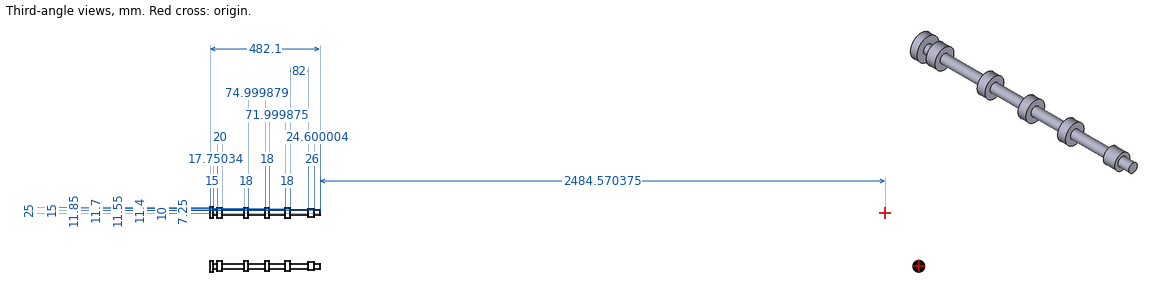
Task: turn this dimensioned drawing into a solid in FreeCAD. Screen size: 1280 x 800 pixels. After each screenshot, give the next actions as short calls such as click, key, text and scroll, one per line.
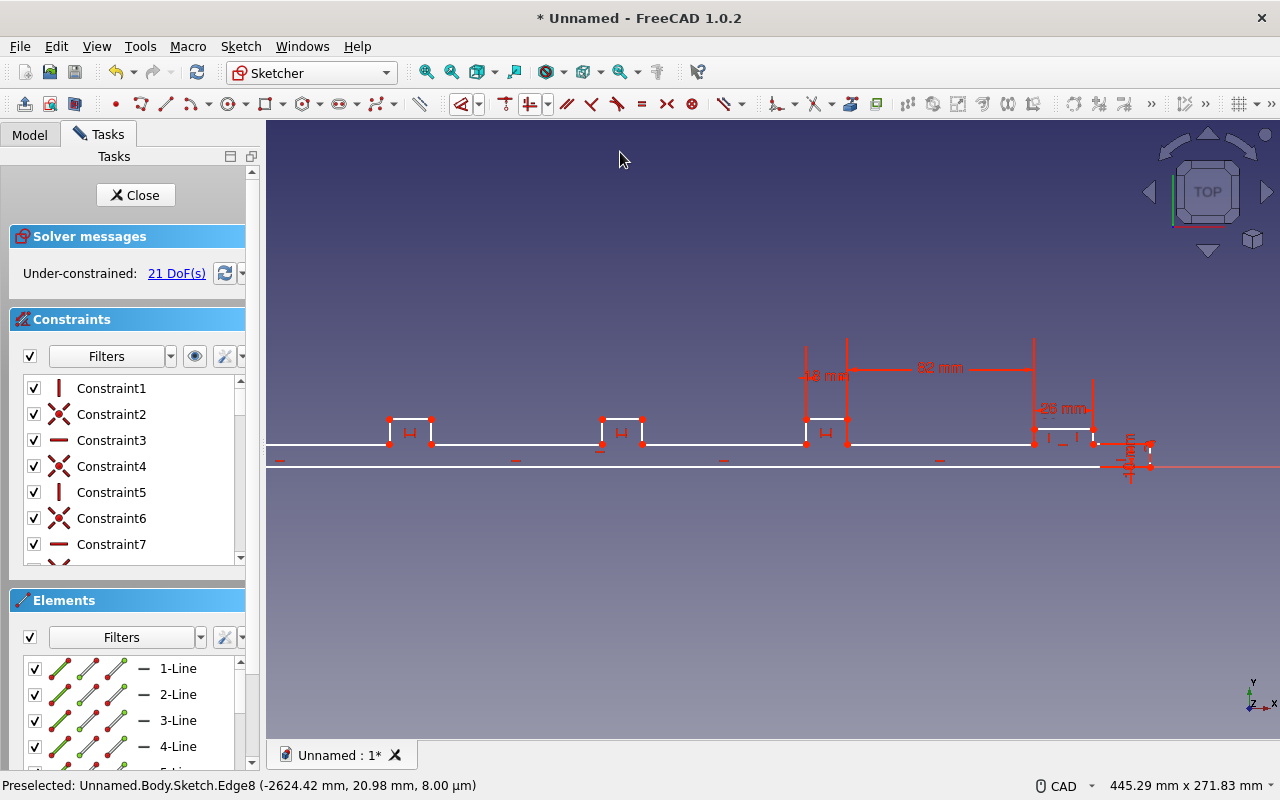
click(630, 419)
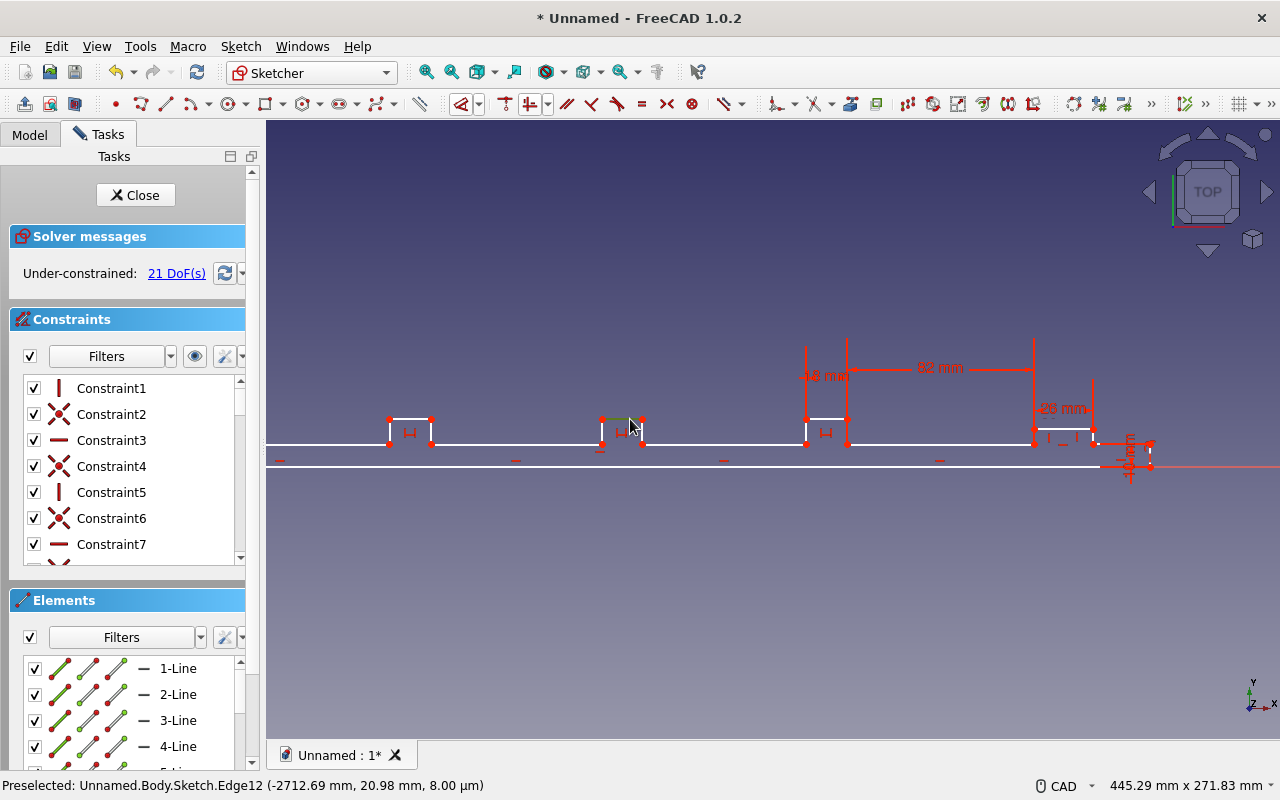
click(478, 104)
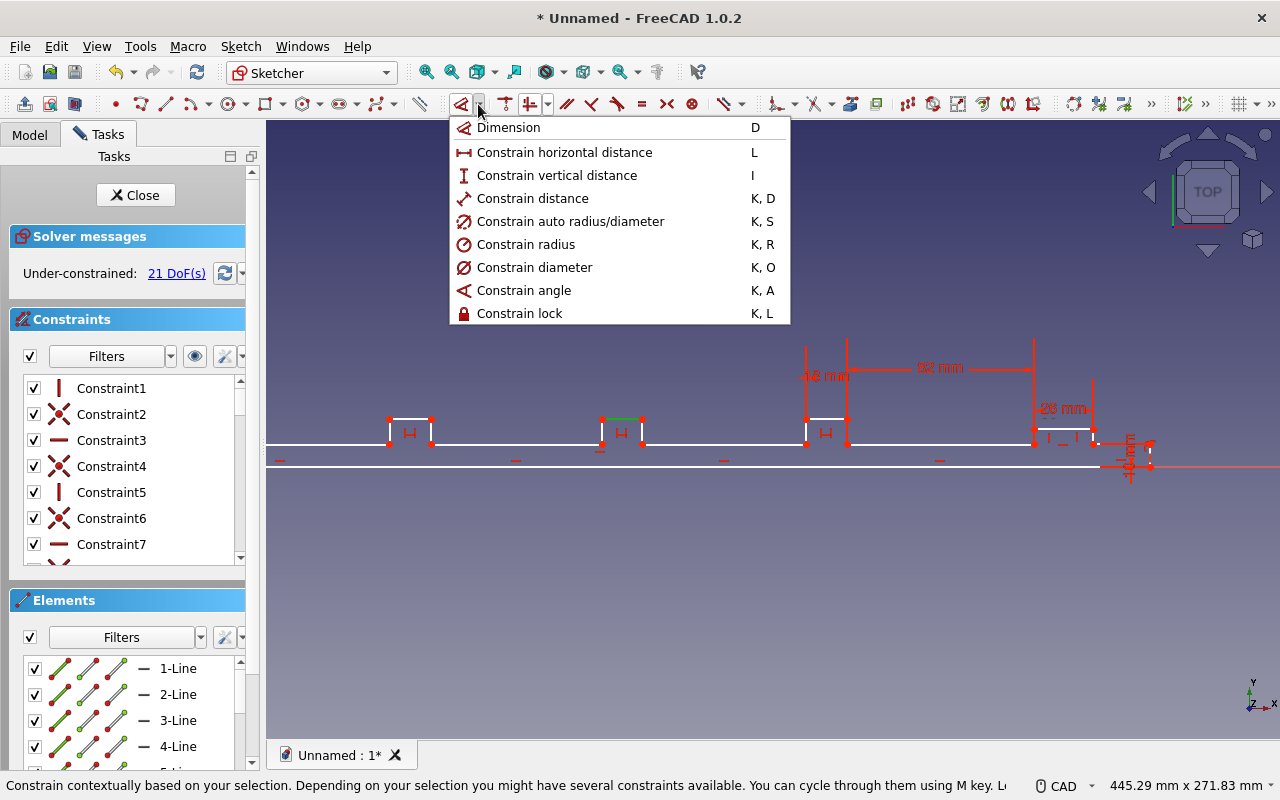
click(620, 152)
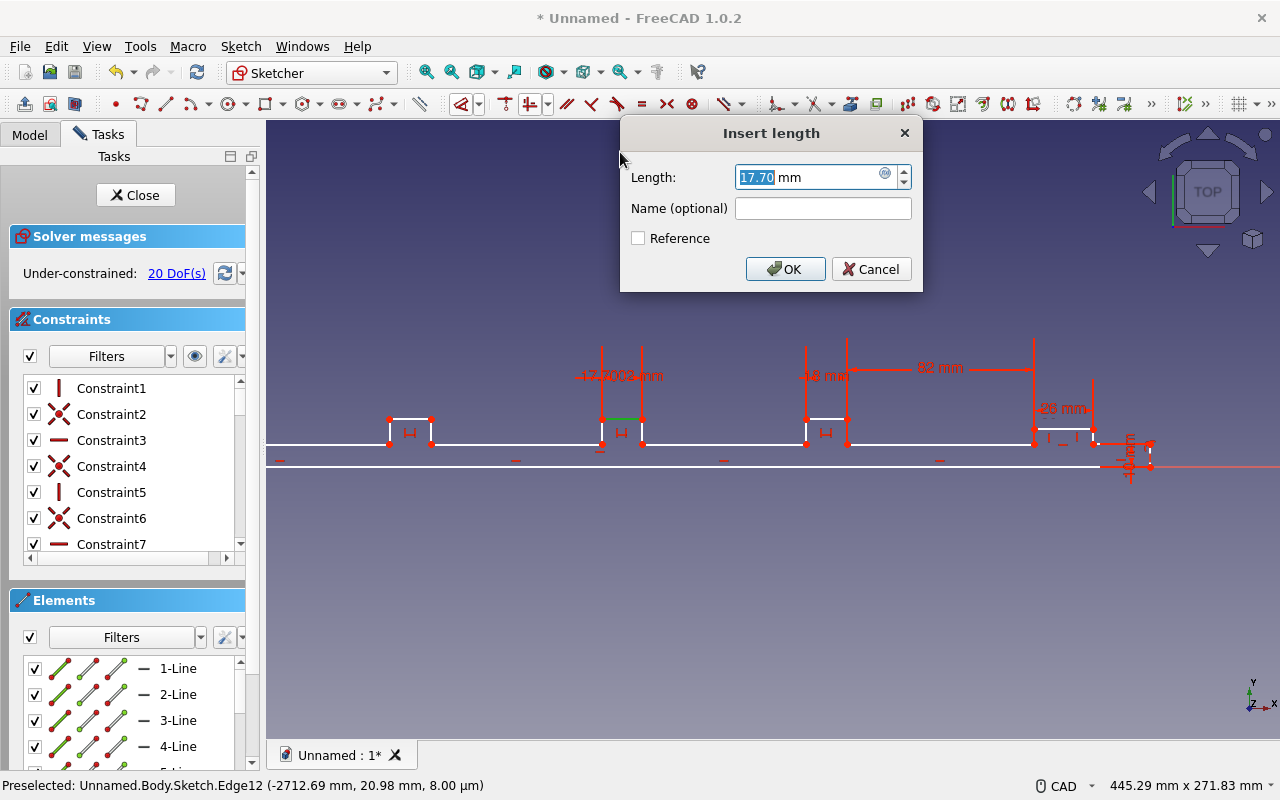
text(18)
key(Return)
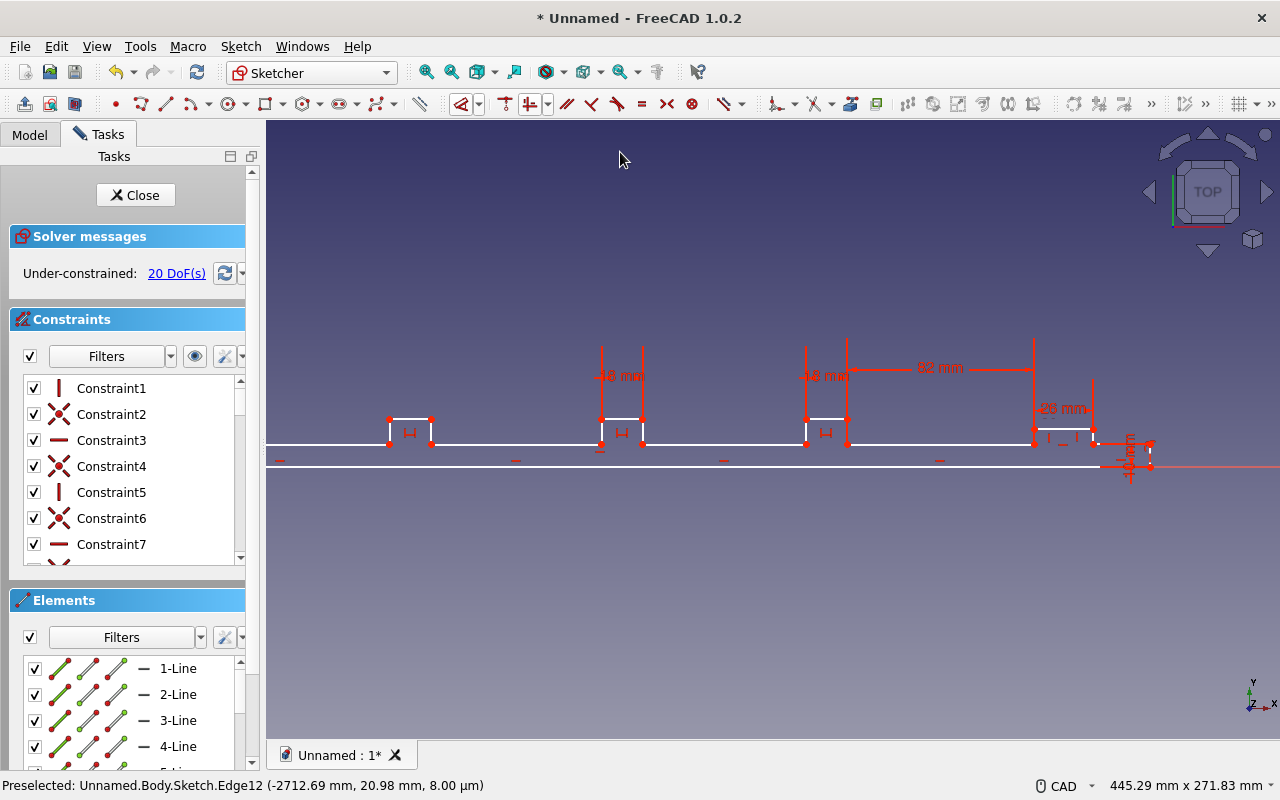
click(419, 419)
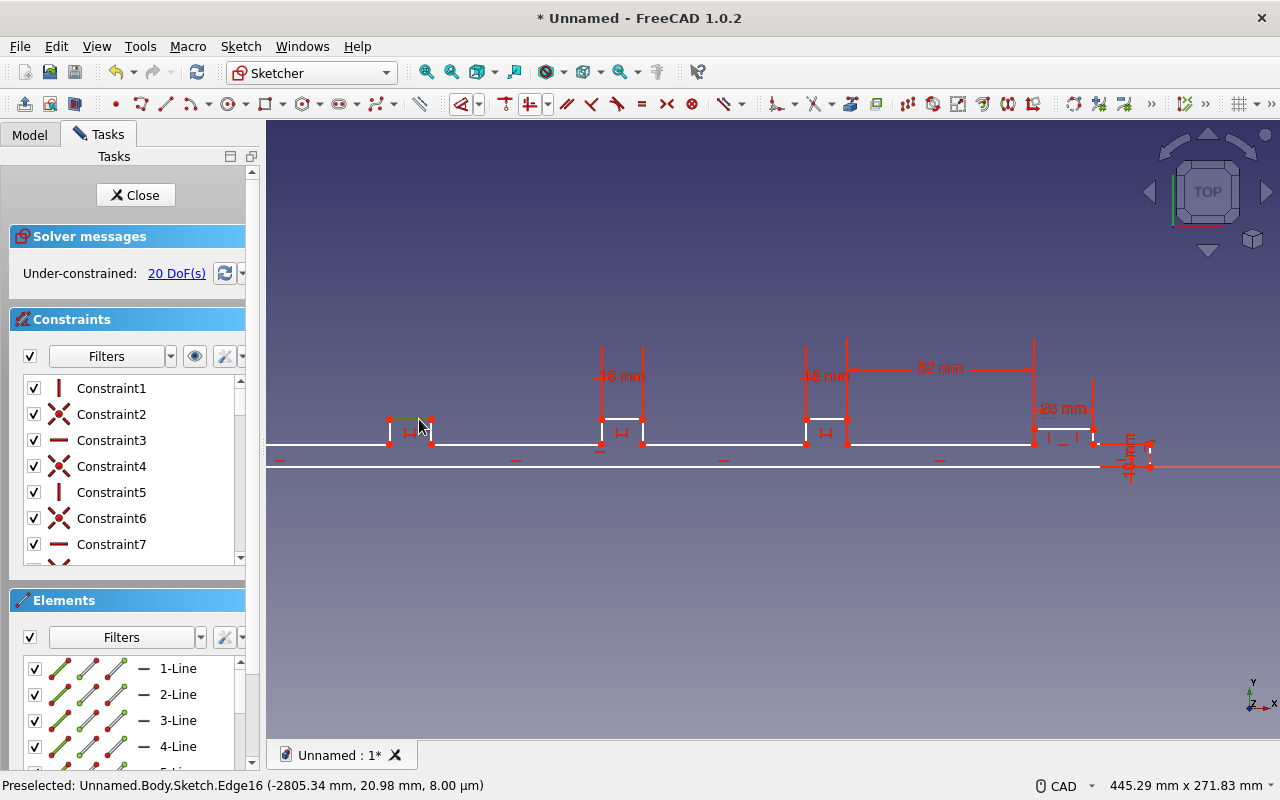
click(478, 104)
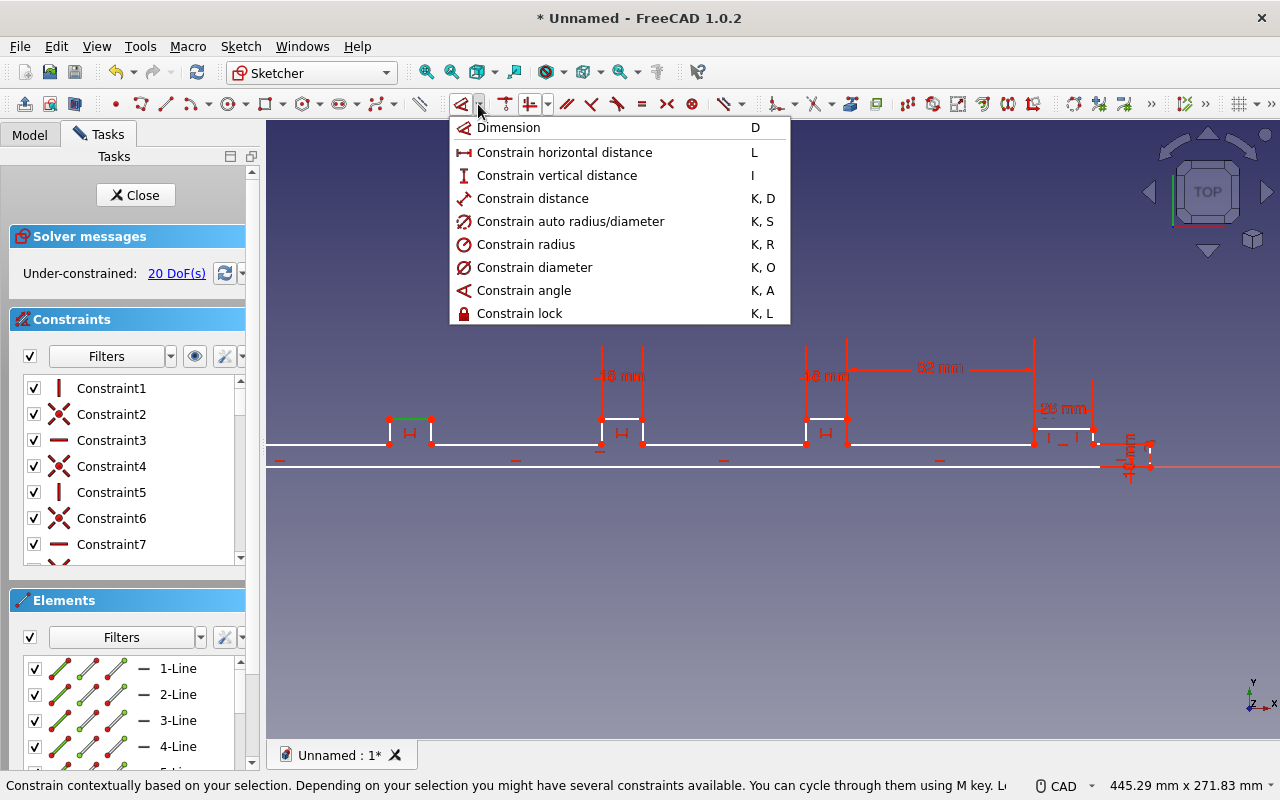
click(620, 152)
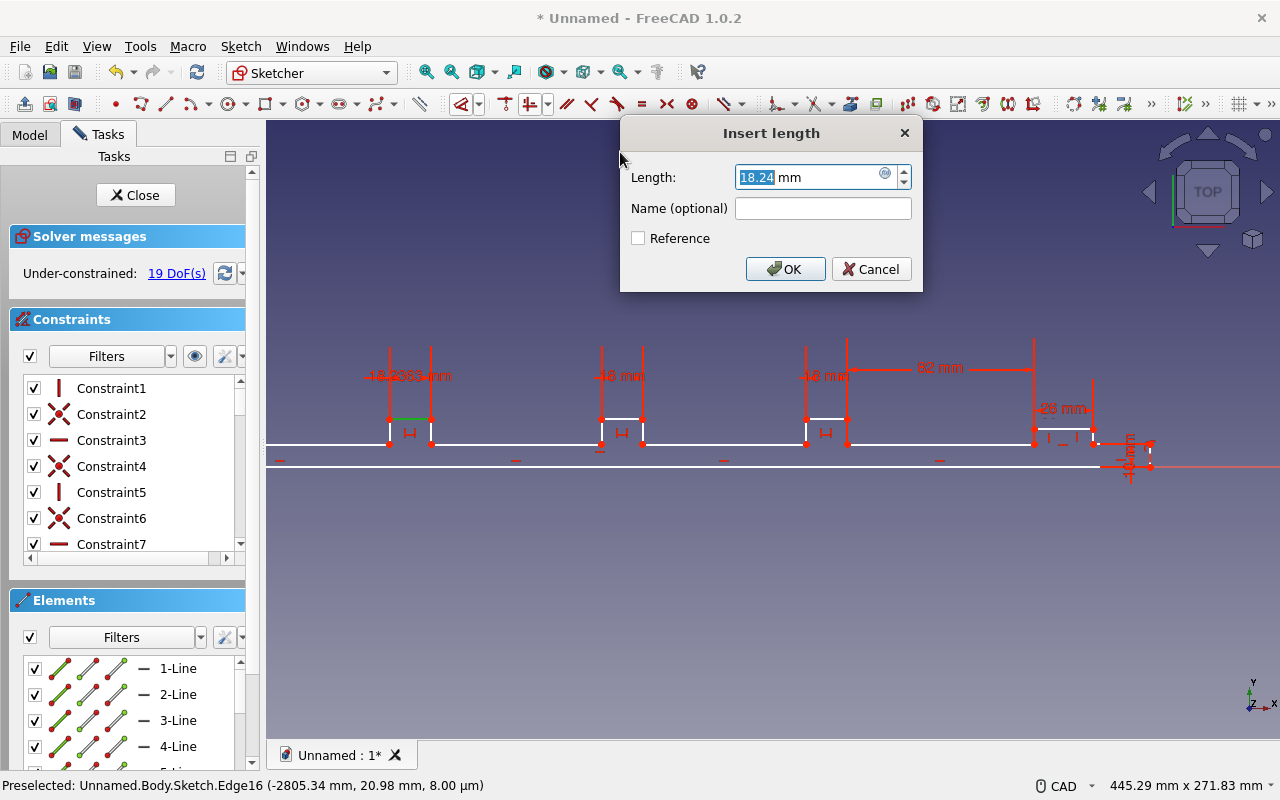
text(18)
key(Return)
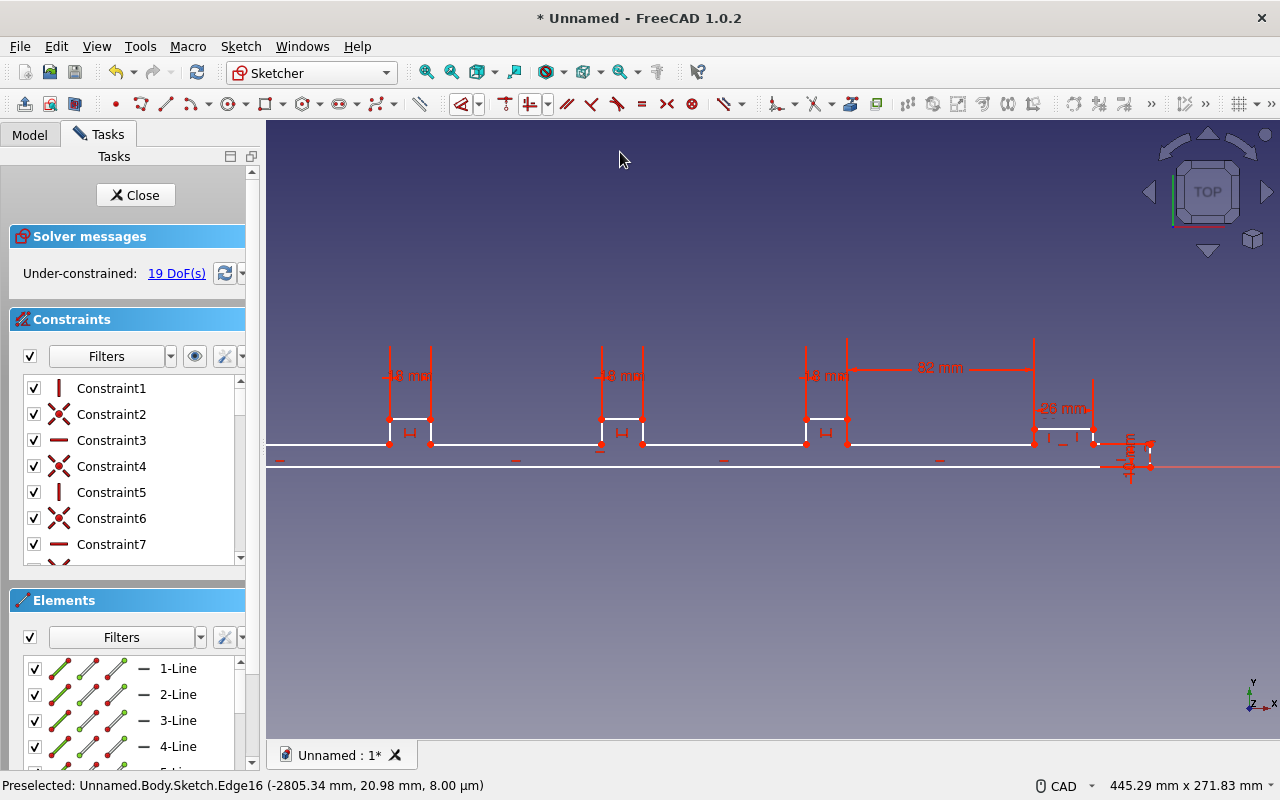
scroll(831, 418, down, 3)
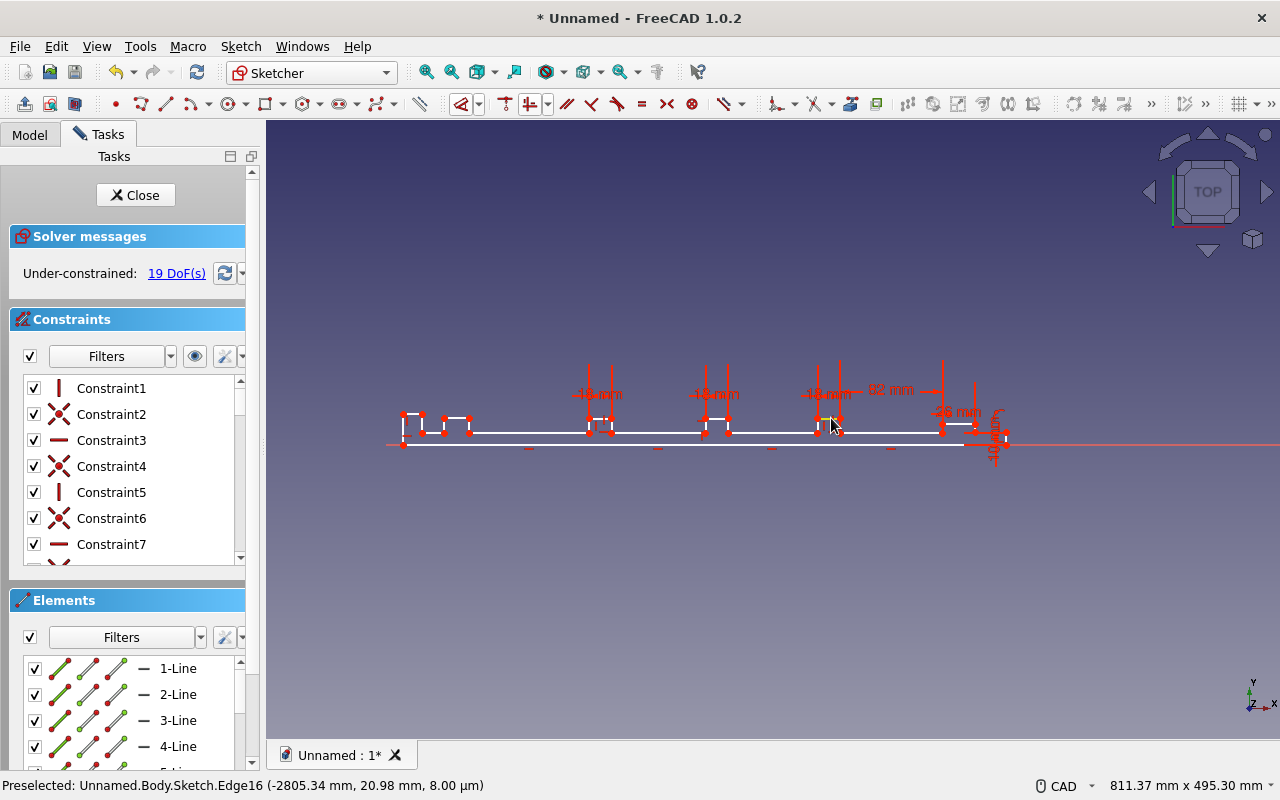
scroll(462, 418, up, 4)